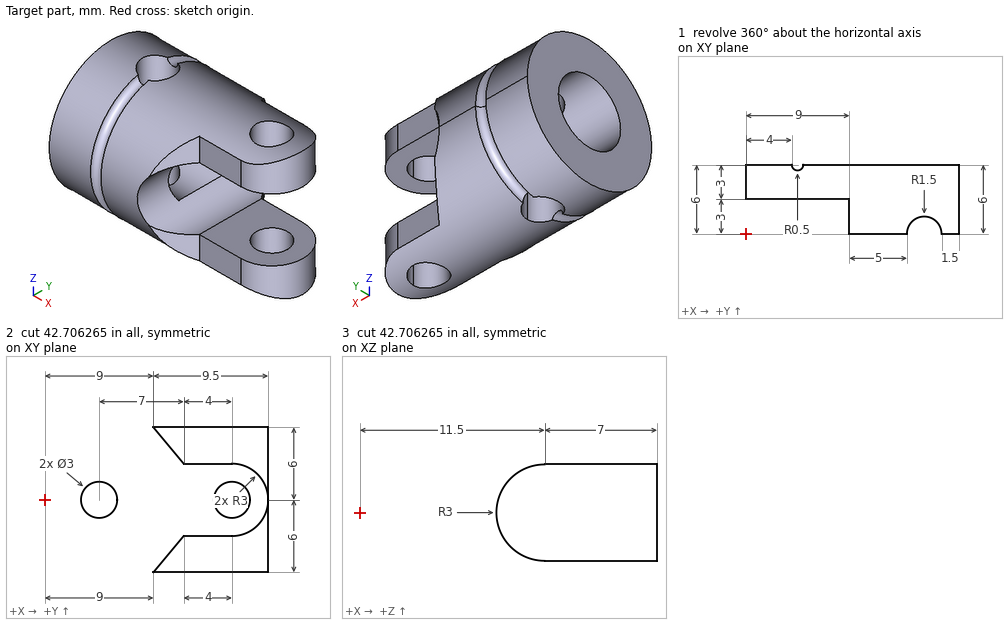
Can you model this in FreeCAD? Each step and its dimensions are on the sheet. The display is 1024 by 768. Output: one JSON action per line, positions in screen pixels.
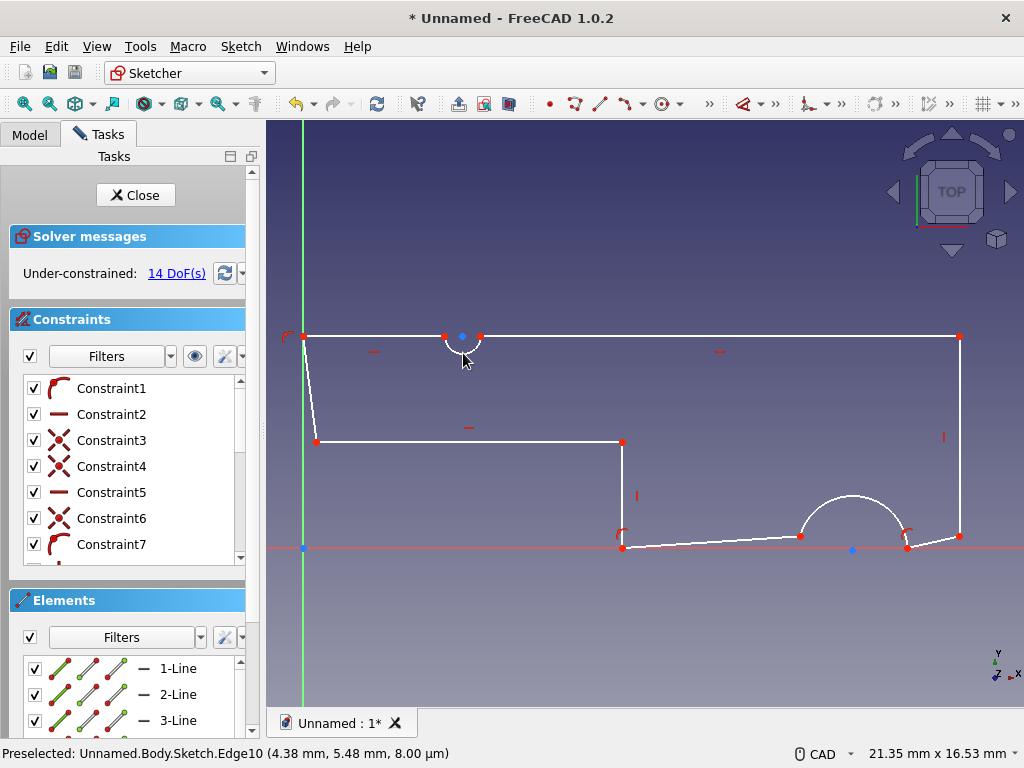
{"action": "scroll", "coordinate": [313, 411], "scroll_direction": "up", "scroll_amount": 2}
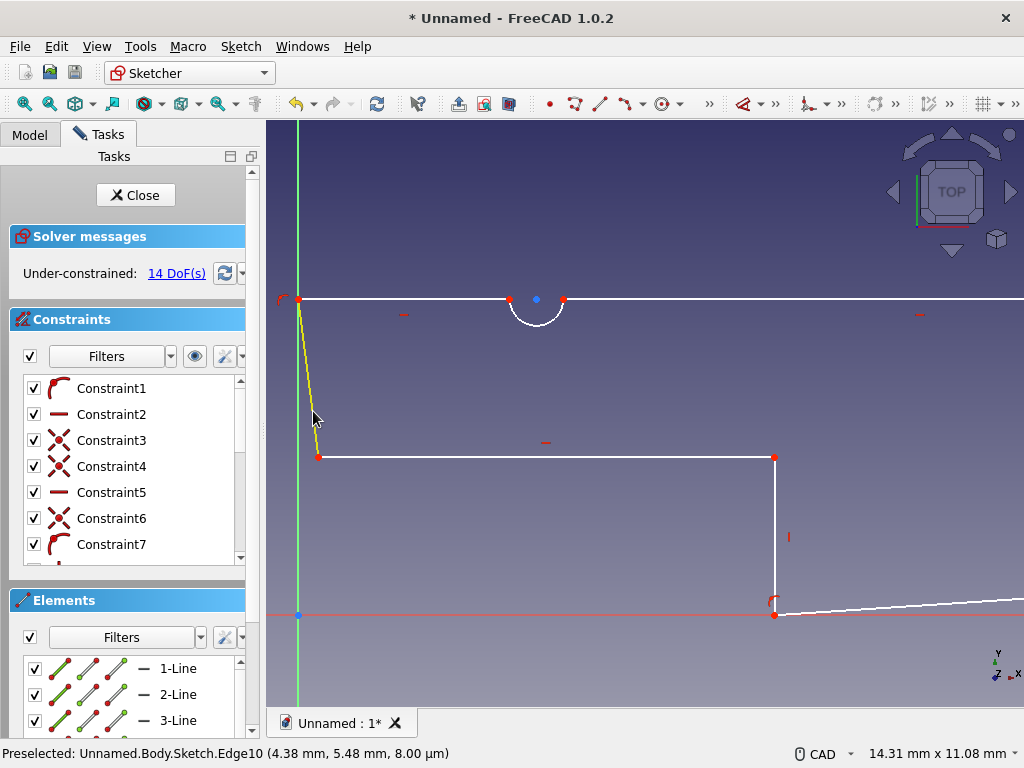
{"action": "left_click", "coordinate": [312, 410]}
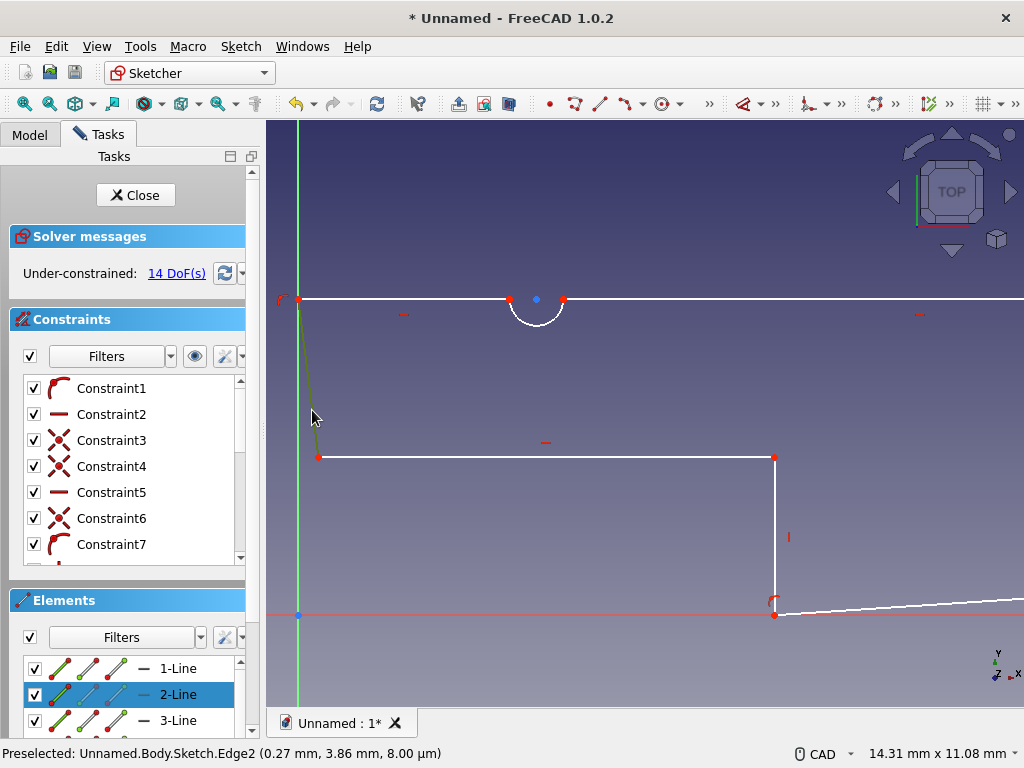
{"action": "key", "text": "v"}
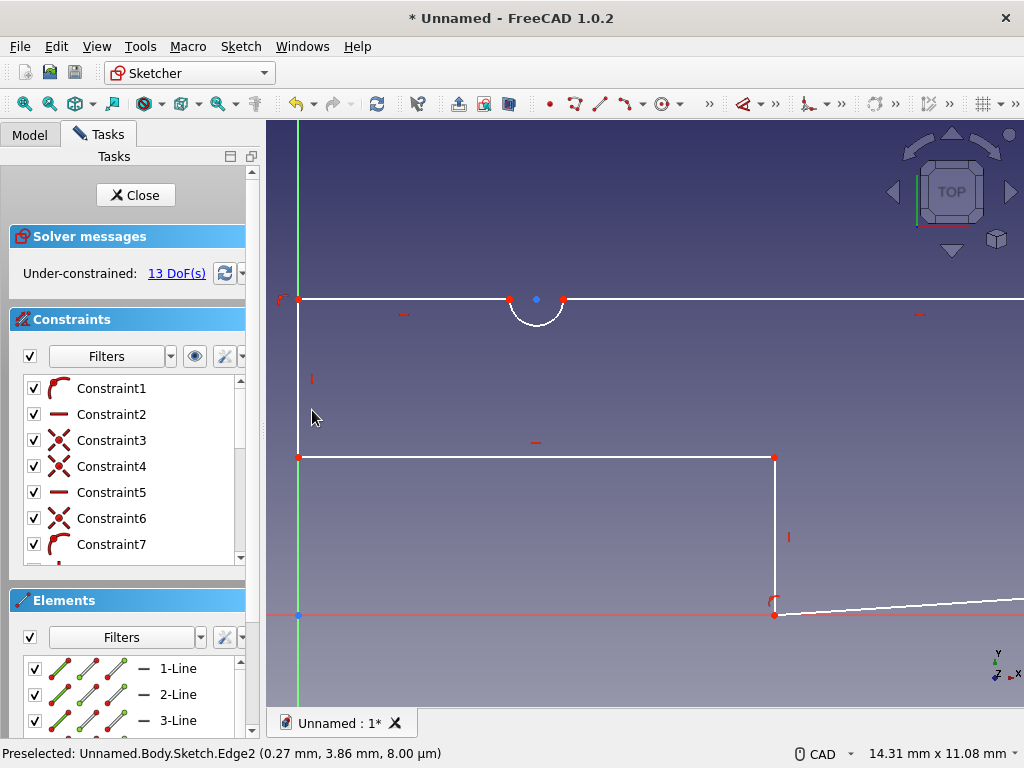
{"action": "left_click", "coordinate": [828, 612]}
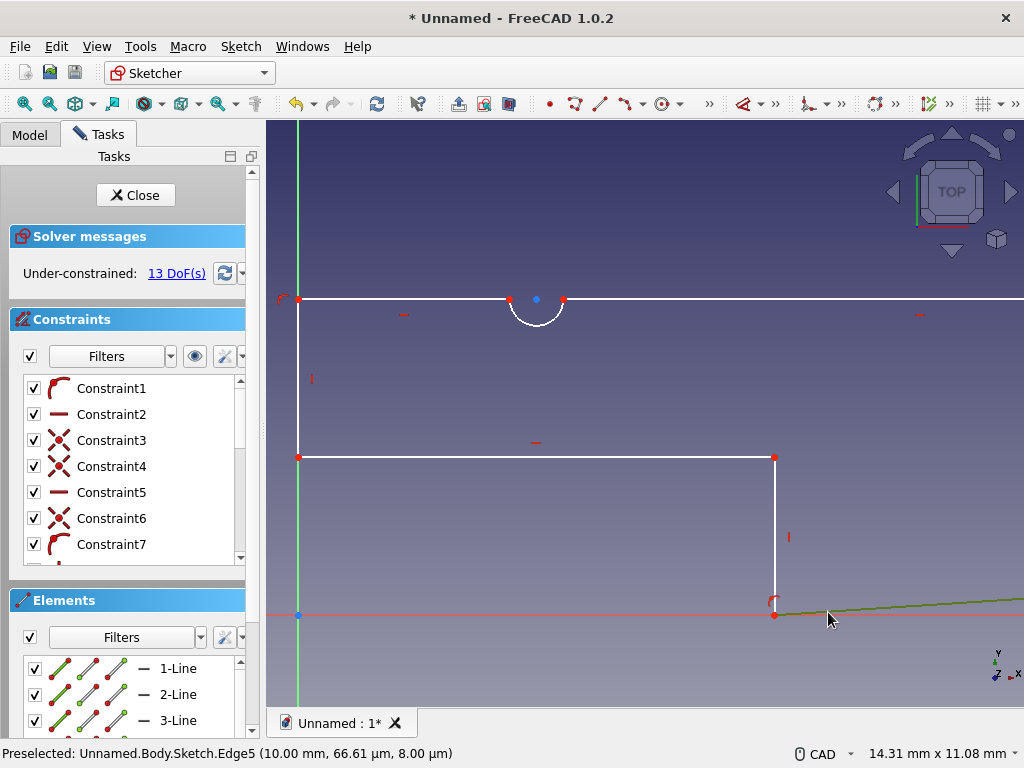
{"action": "key", "text": "h"}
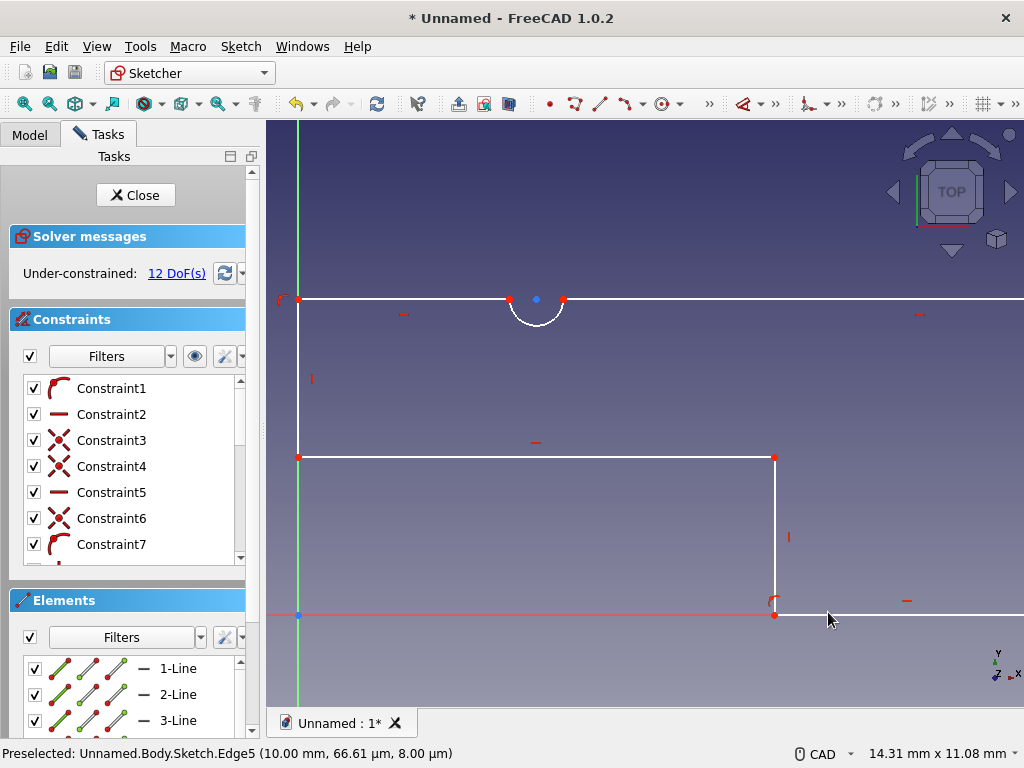
{"action": "scroll", "coordinate": [404, 379], "scroll_direction": "down", "scroll_amount": 4}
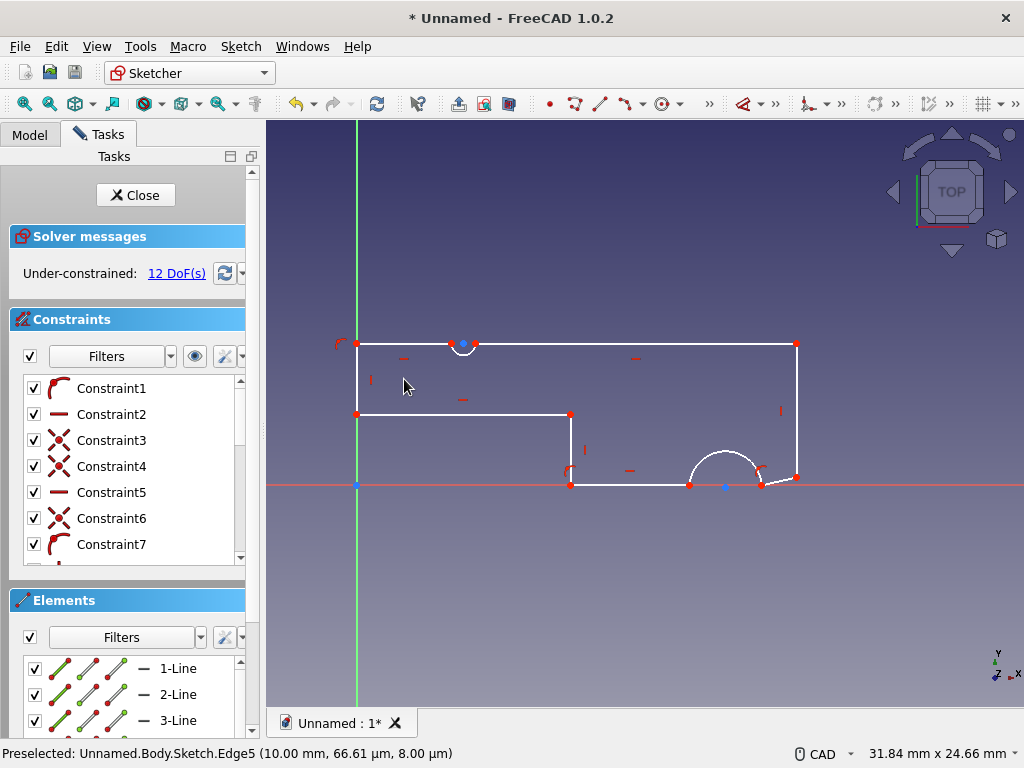
{"action": "scroll", "coordinate": [786, 480], "scroll_direction": "up", "scroll_amount": 5}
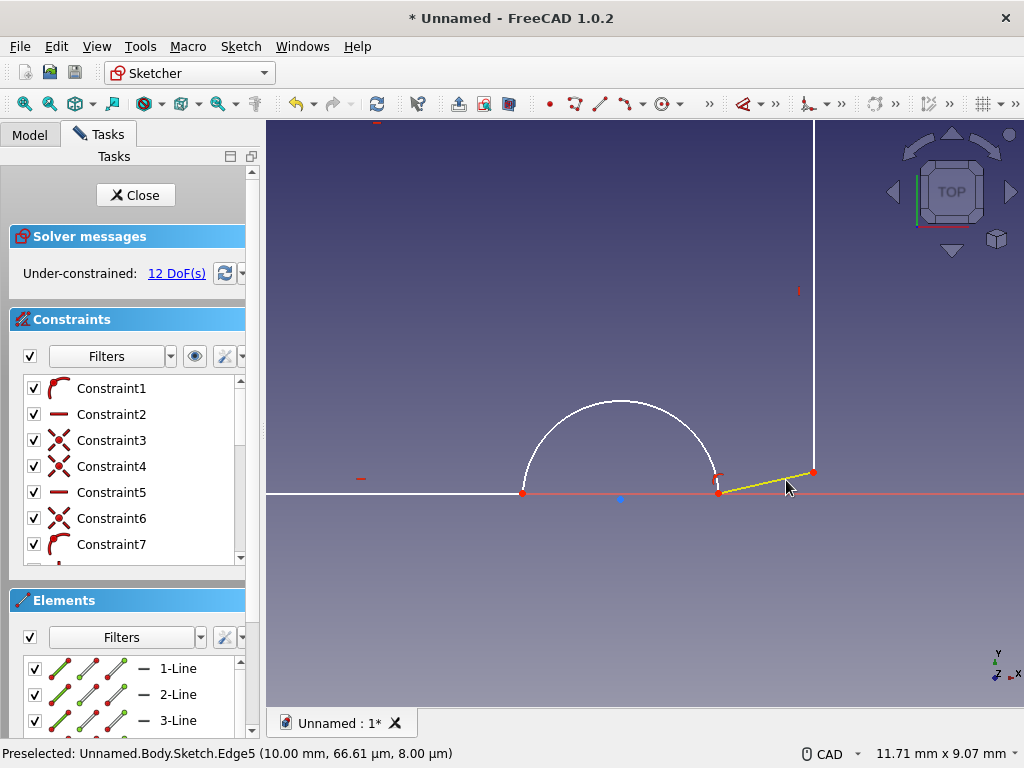
{"action": "left_click", "coordinate": [785, 479]}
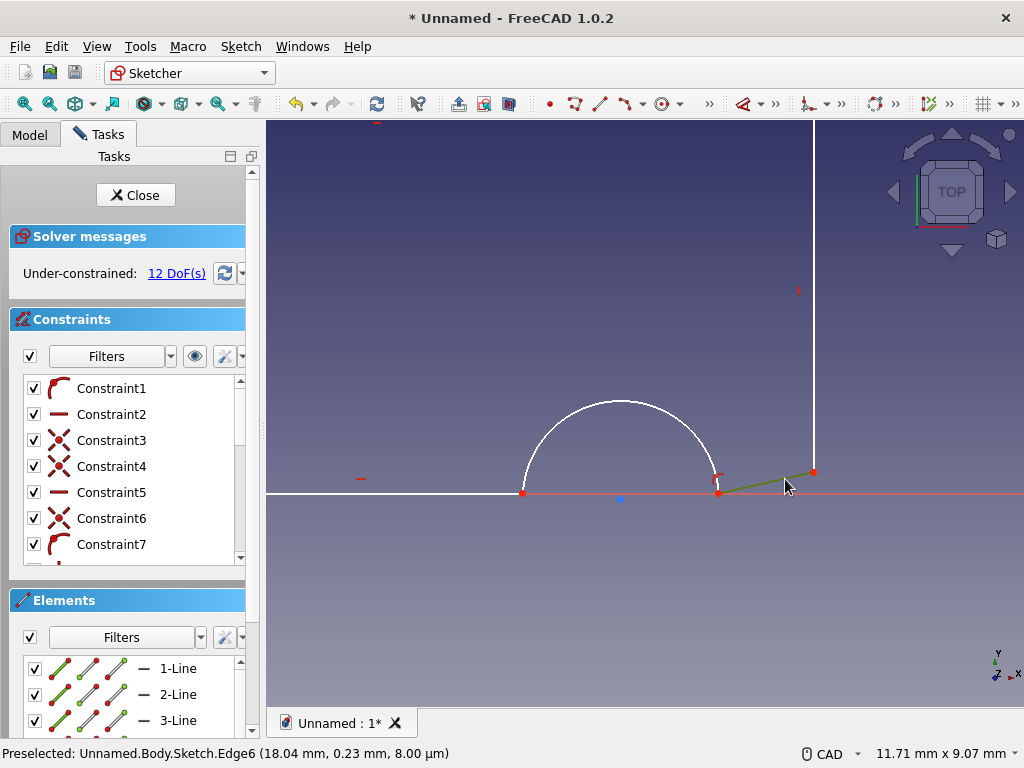
{"action": "key", "text": "h"}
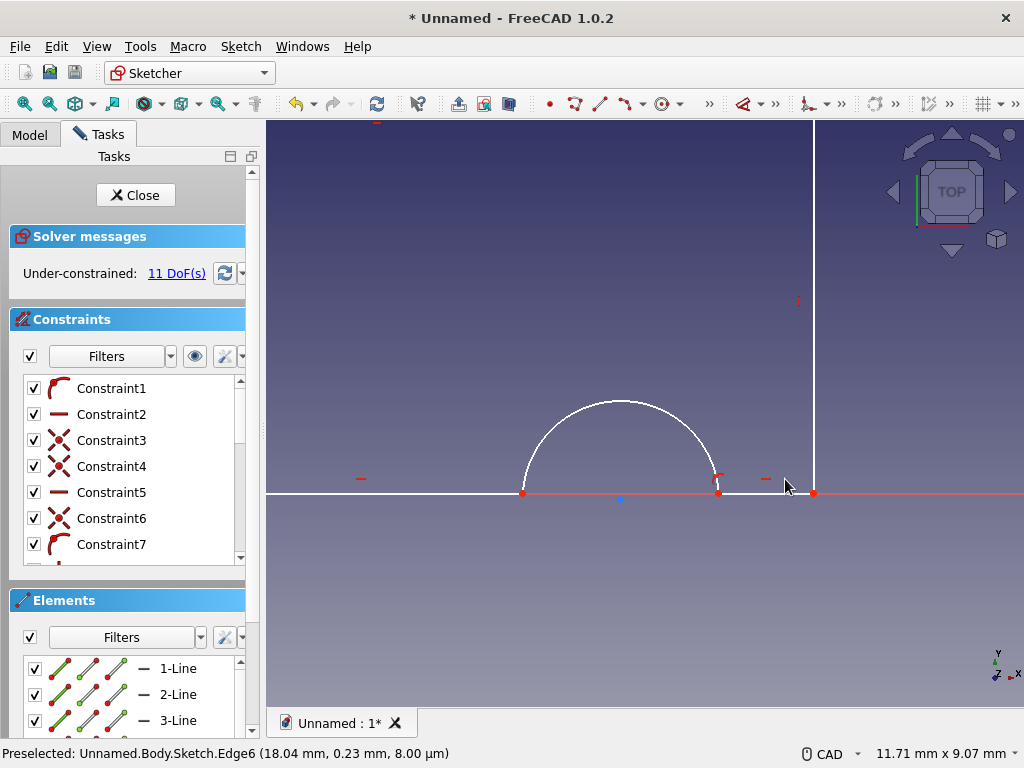
{"action": "left_click", "coordinate": [621, 499]}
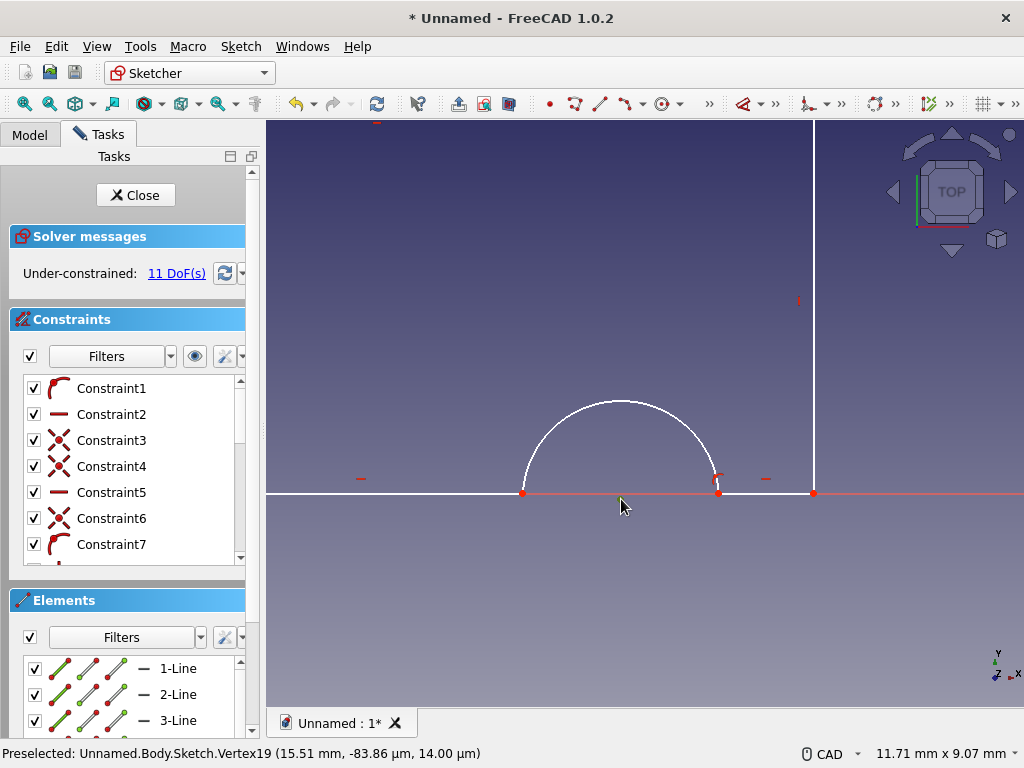
{"action": "left_click", "coordinate": [576, 494]}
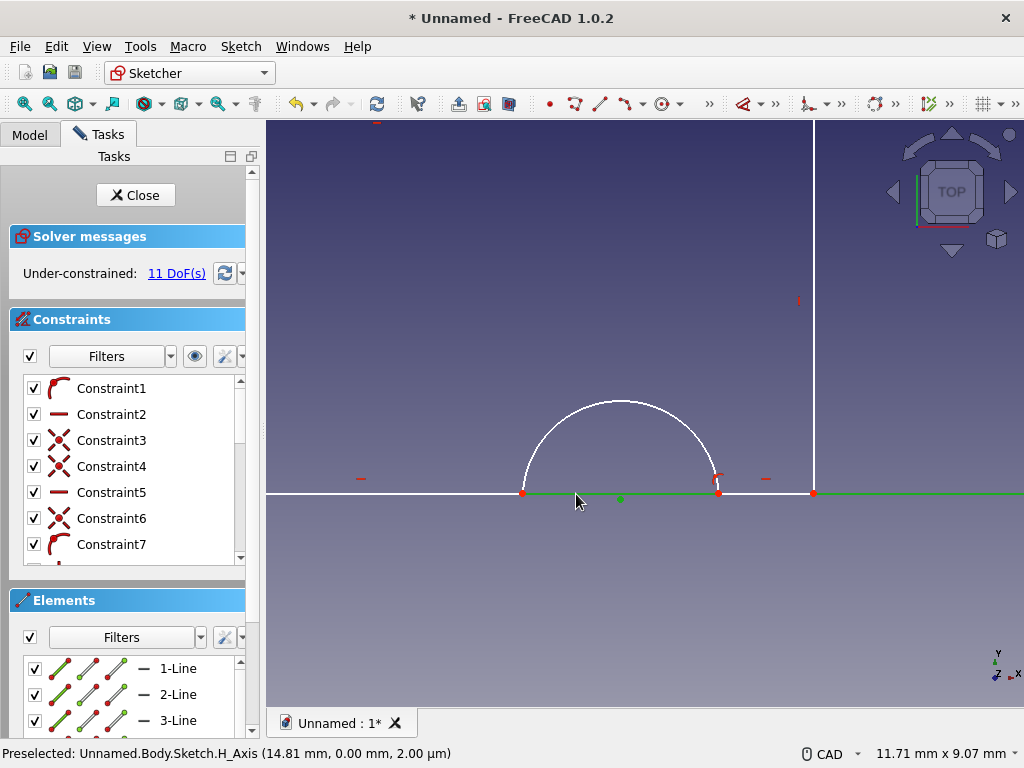
{"action": "key", "text": "c"}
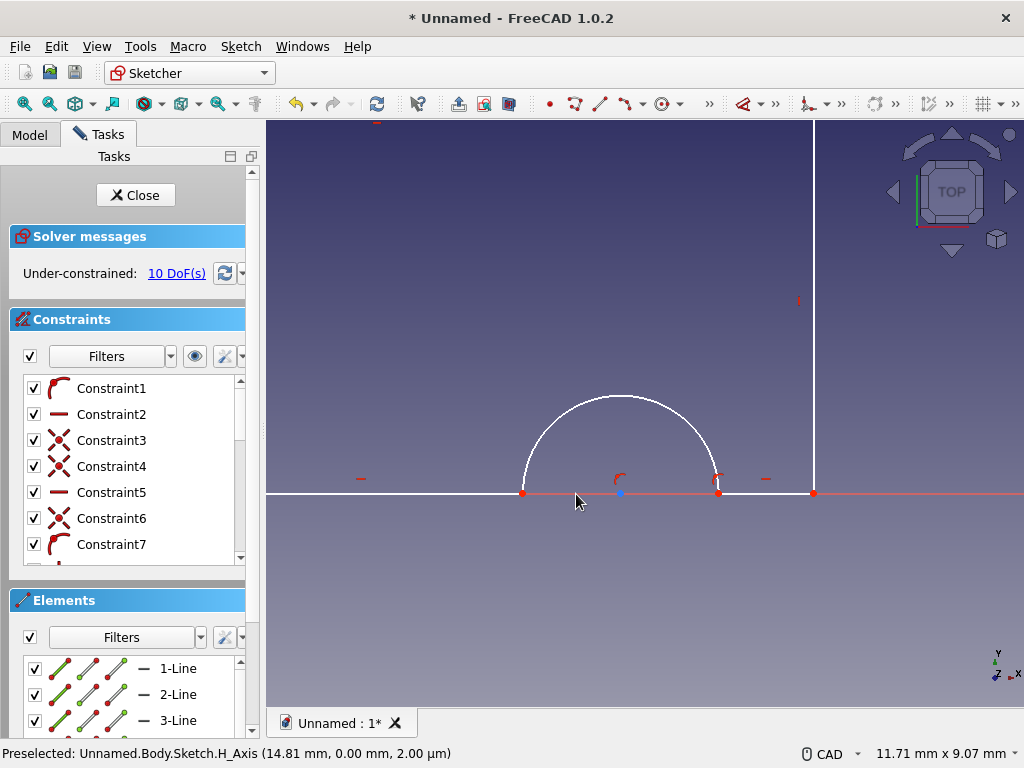
{"action": "left_click", "coordinate": [742, 104]}